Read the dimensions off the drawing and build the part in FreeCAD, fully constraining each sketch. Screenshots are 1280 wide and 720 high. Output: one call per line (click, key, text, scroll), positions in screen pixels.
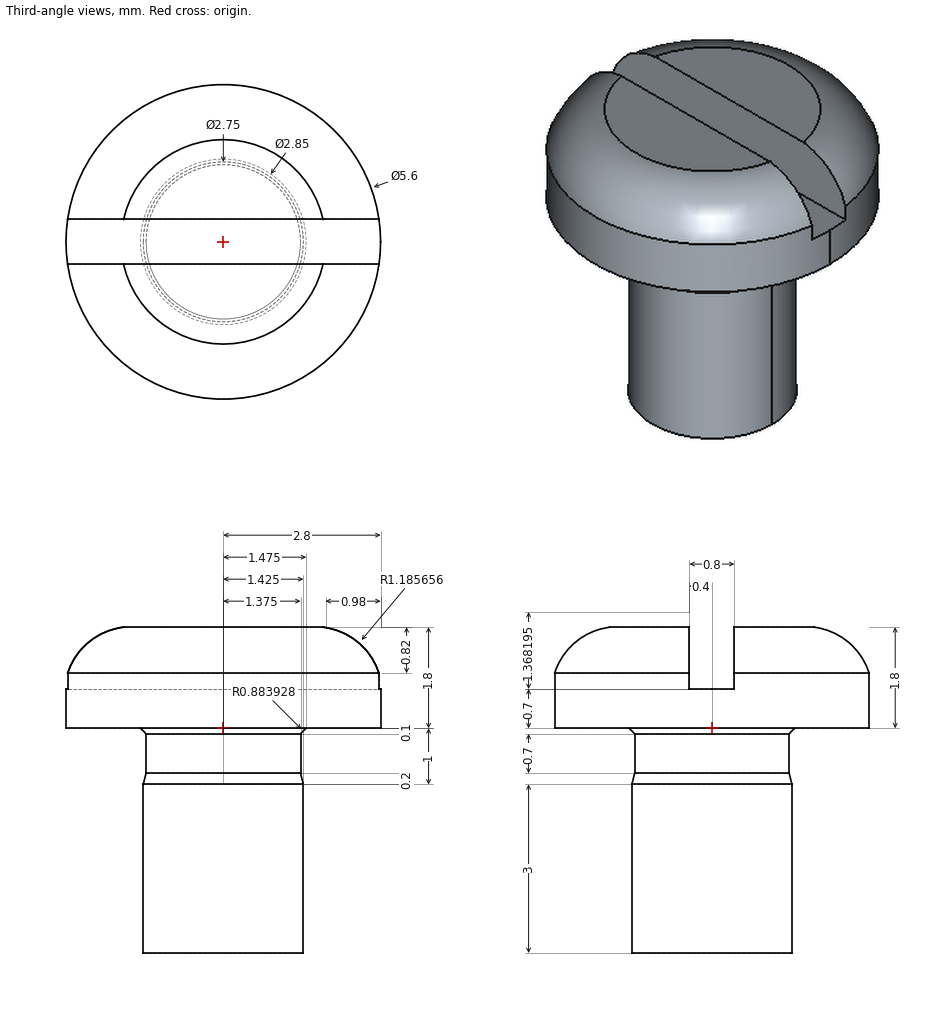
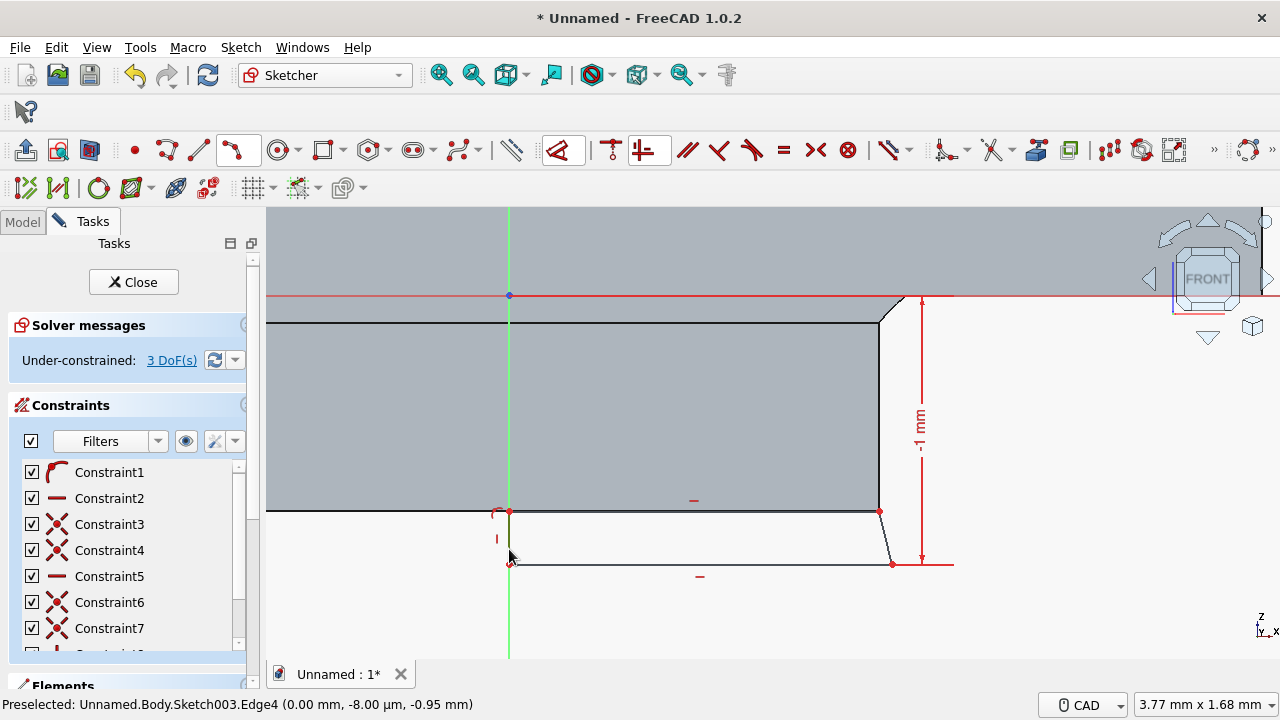
key(i)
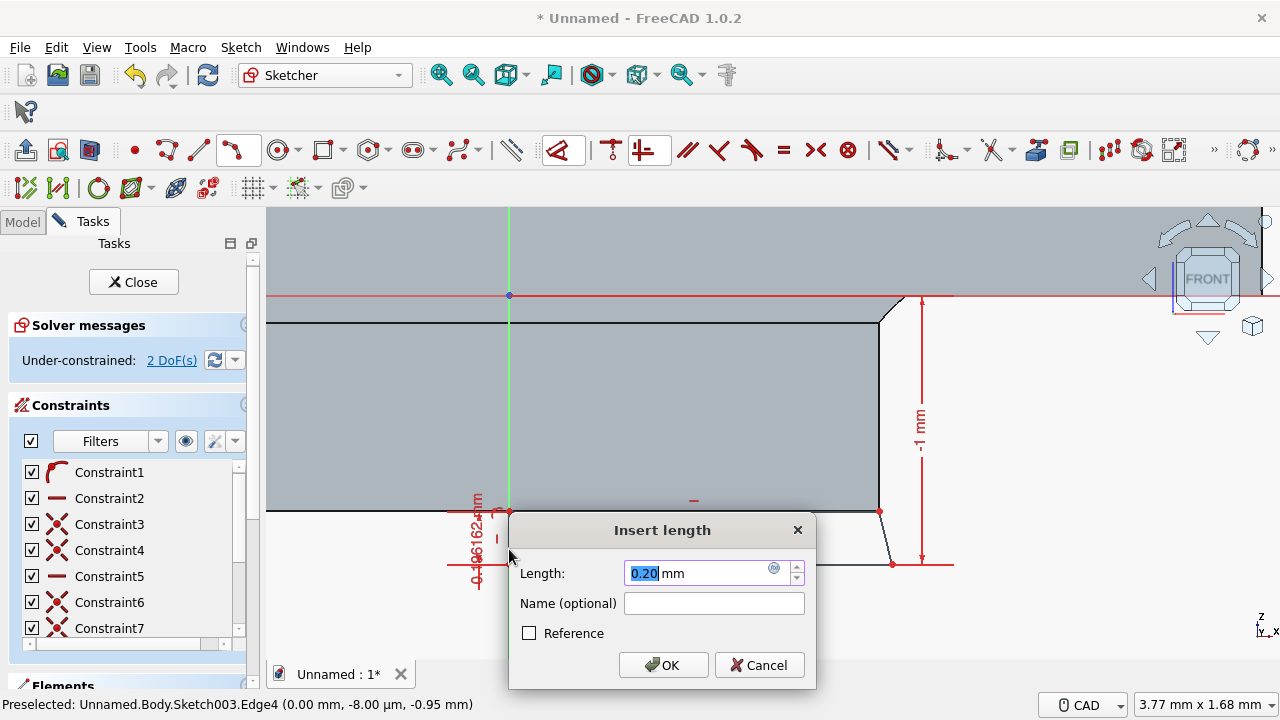
text(0.2)
key(Return)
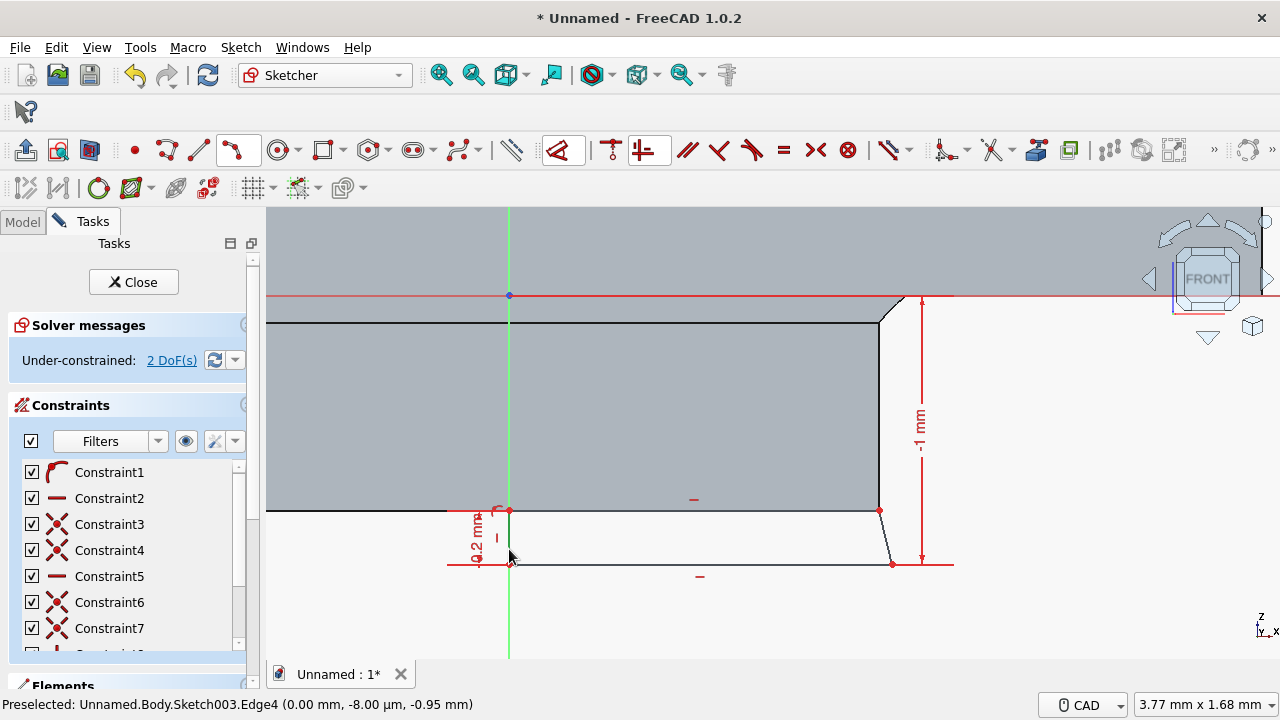
click(620, 511)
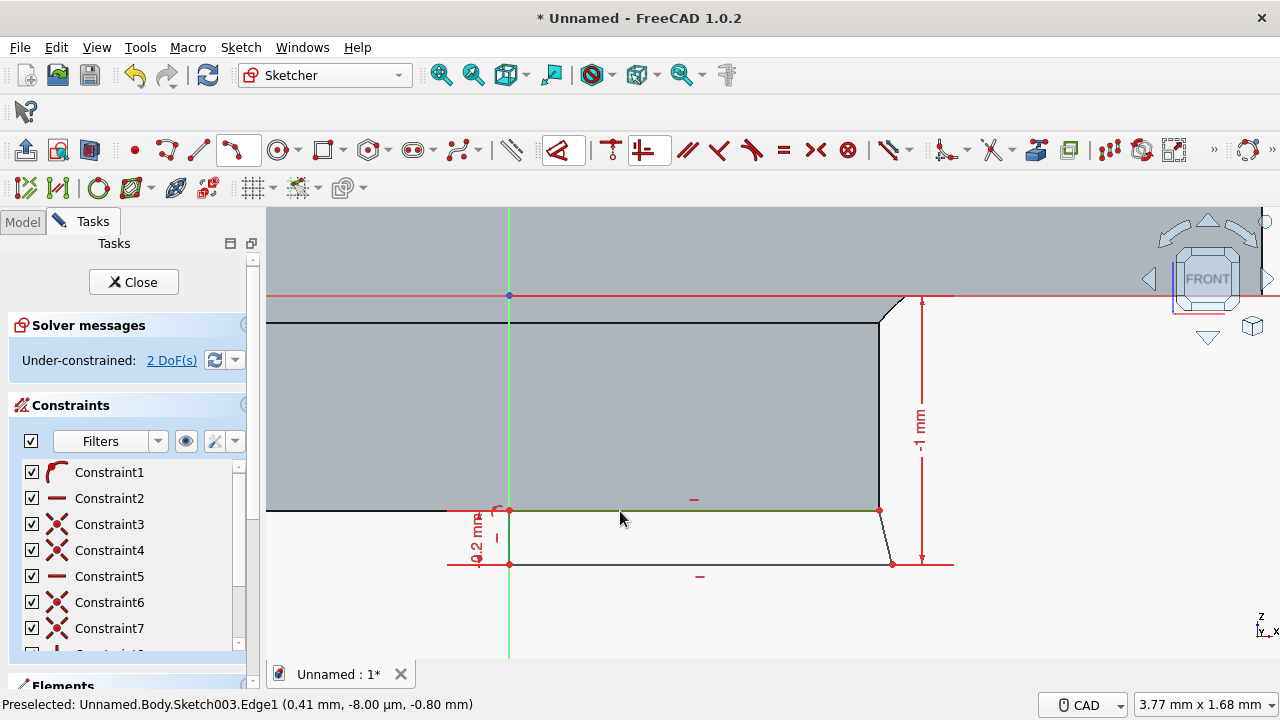
key(l)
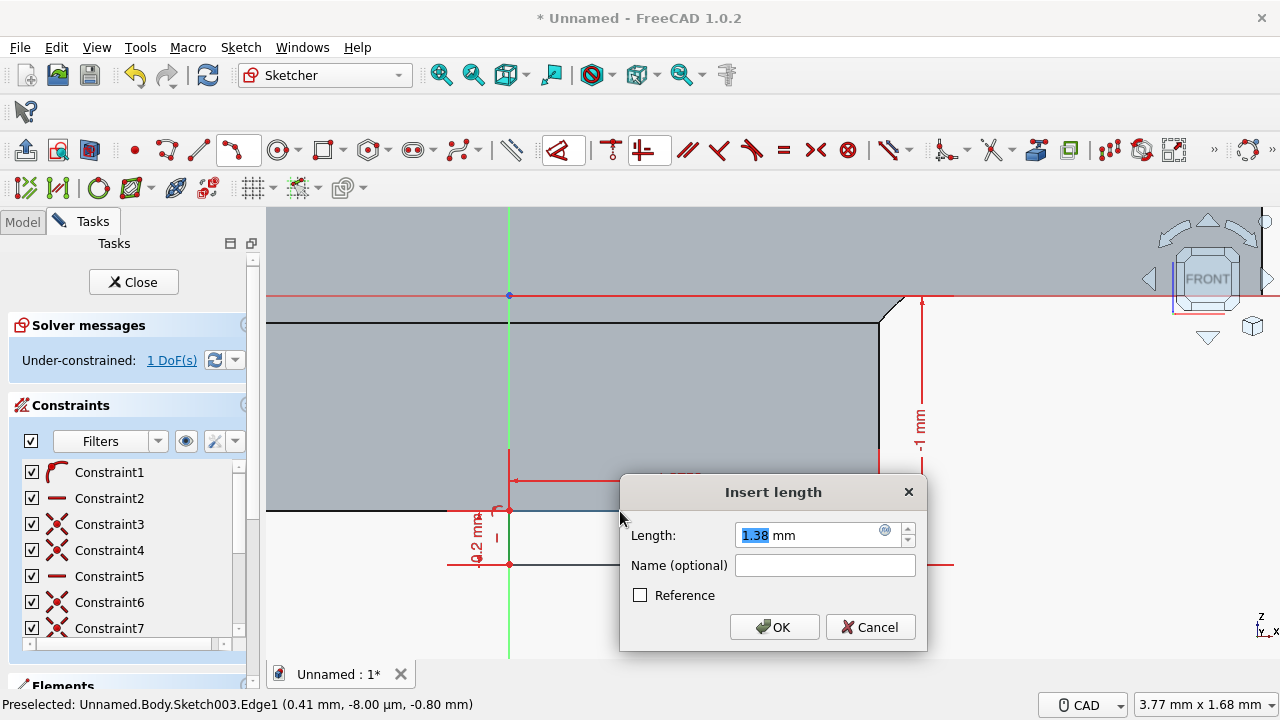
text(1.375)
key(Return)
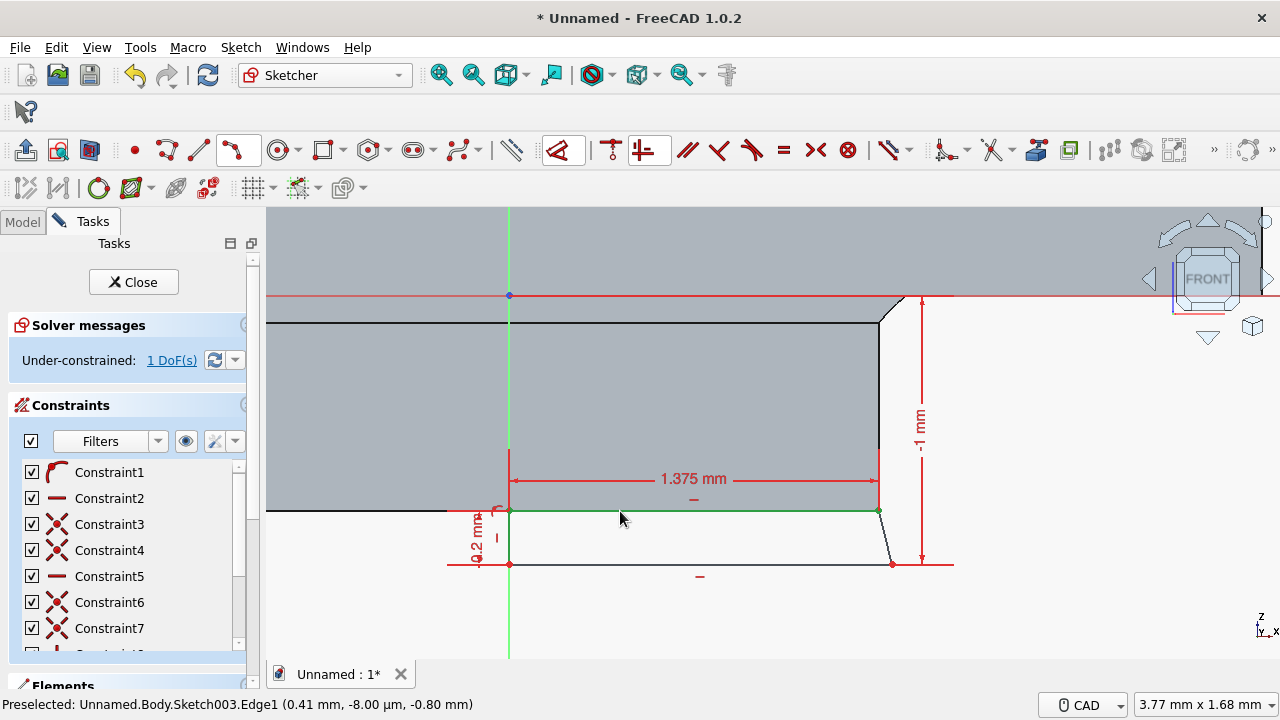
click(777, 565)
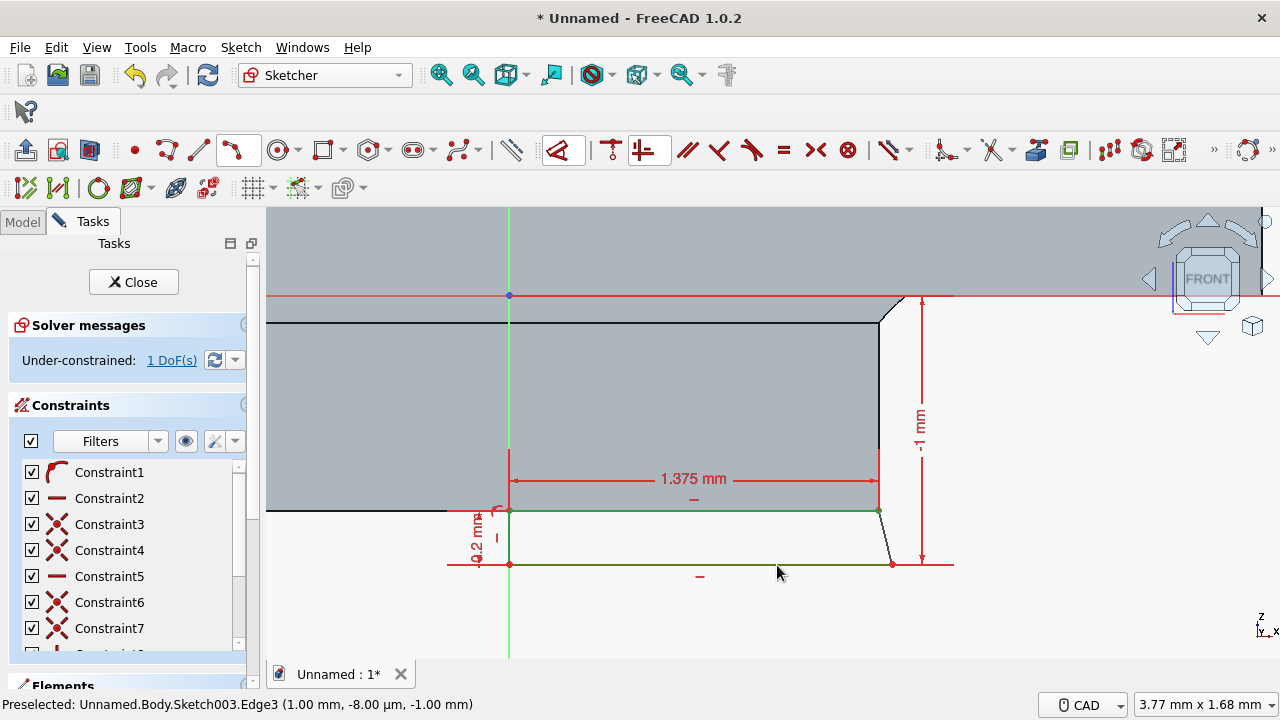
key(l)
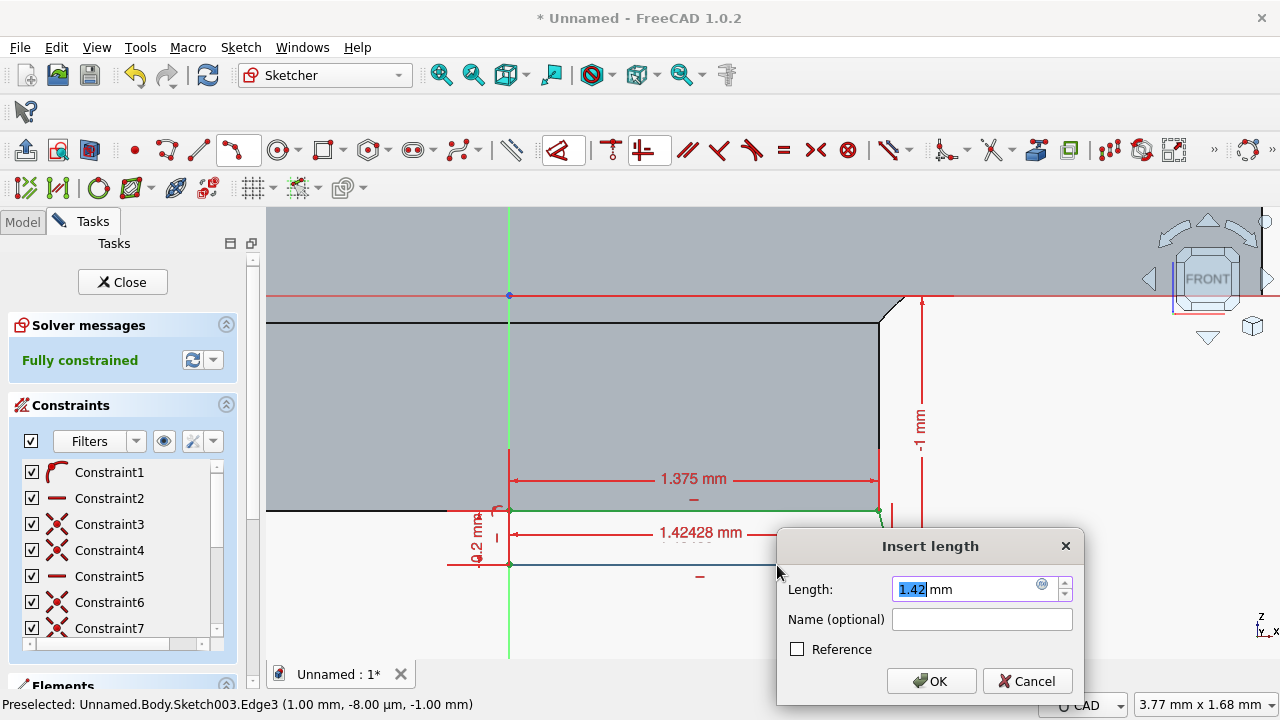
text(1.425)
key(Return)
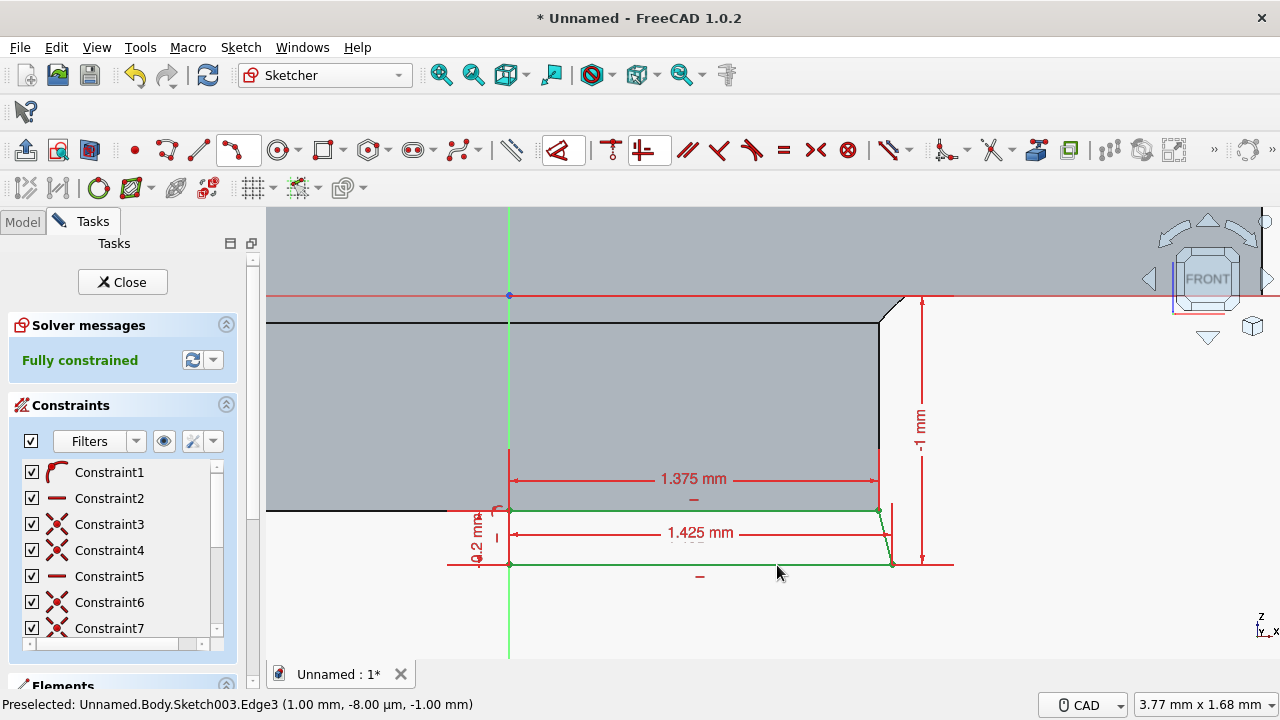
click(123, 282)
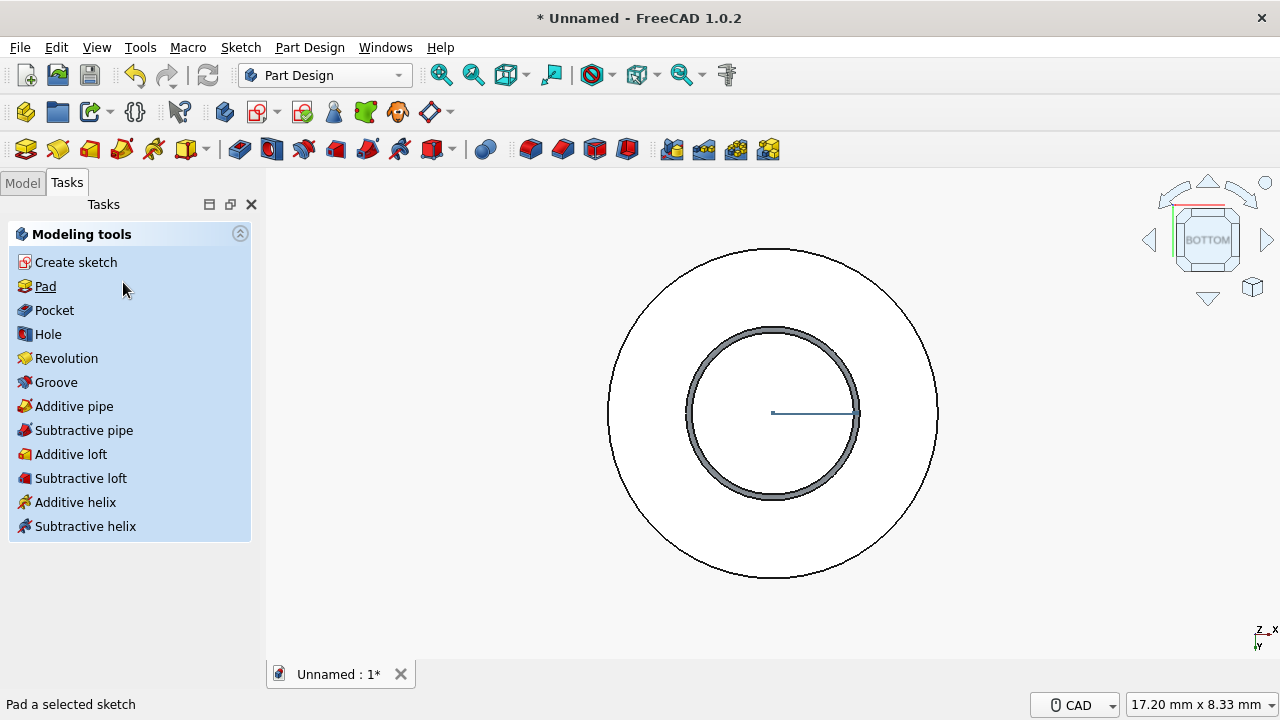
click(58, 150)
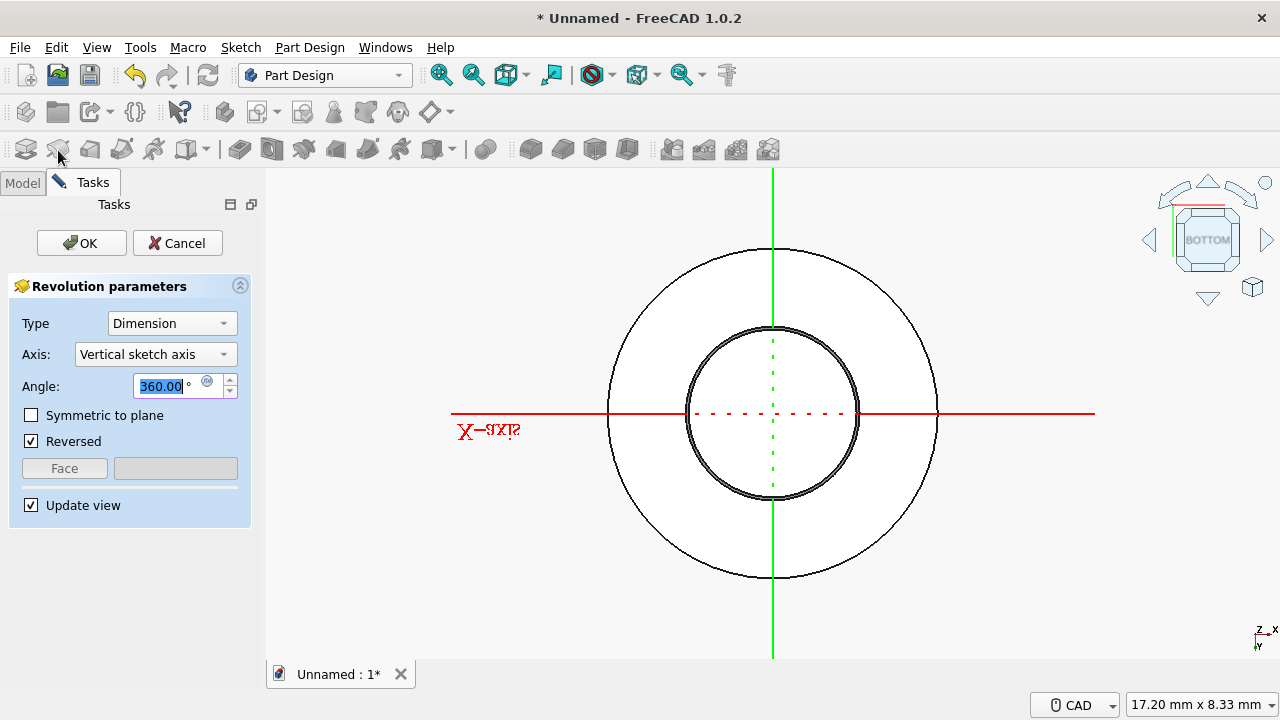
click(82, 243)